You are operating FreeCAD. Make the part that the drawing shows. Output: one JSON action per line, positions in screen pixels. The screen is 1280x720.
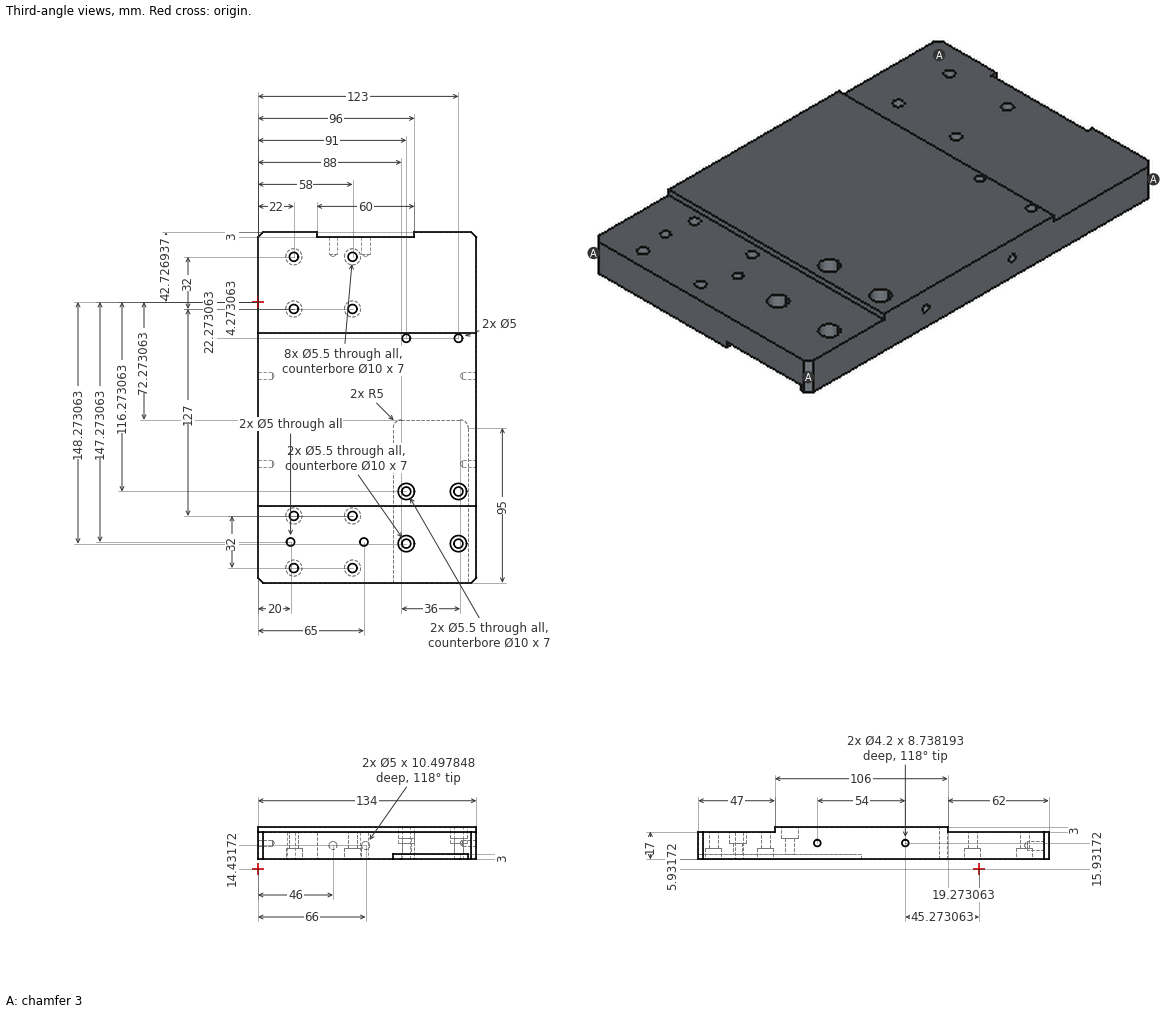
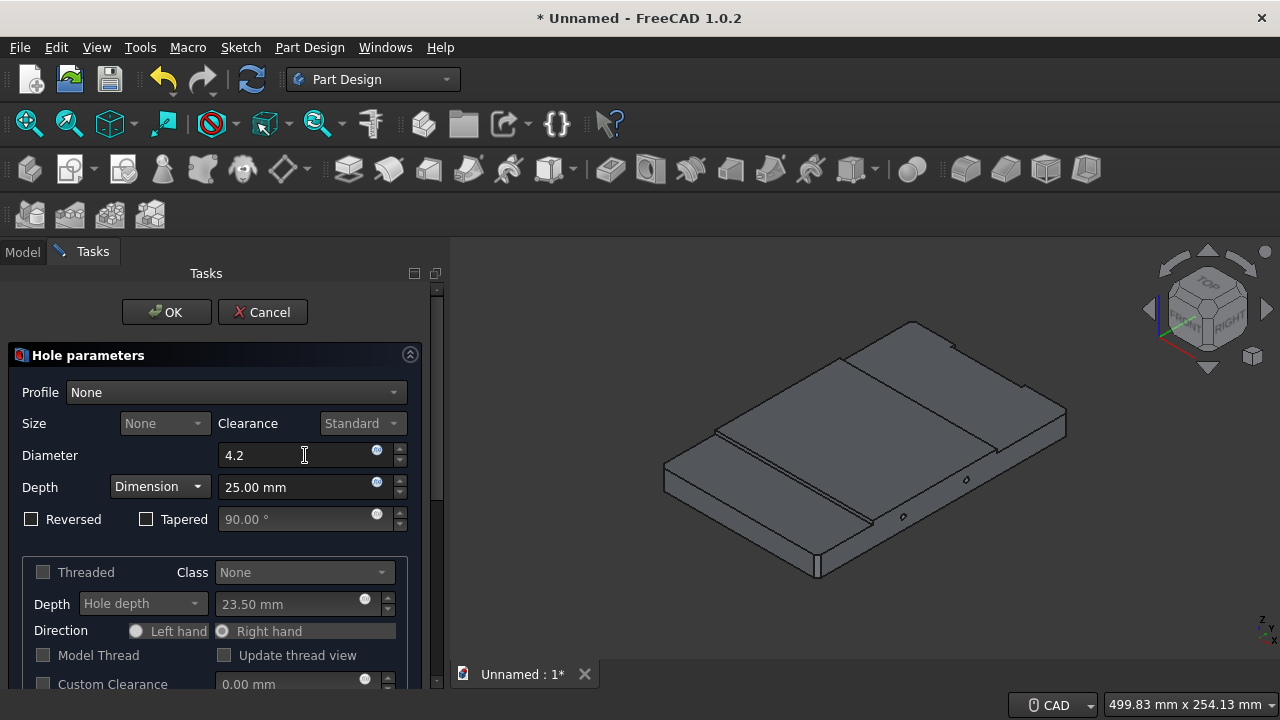
{"action": "triple_click", "coordinate": [305, 487]}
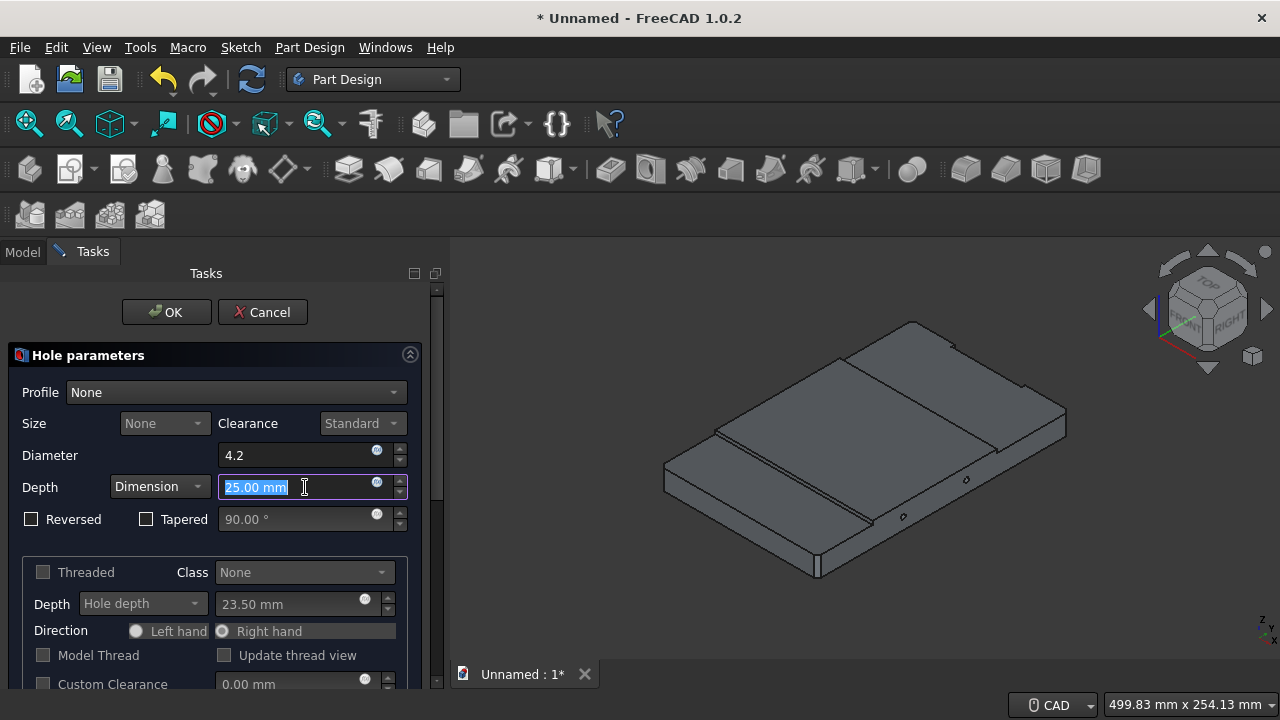
{"action": "type", "text": "8.738193"}
{"action": "key", "text": "Tab"}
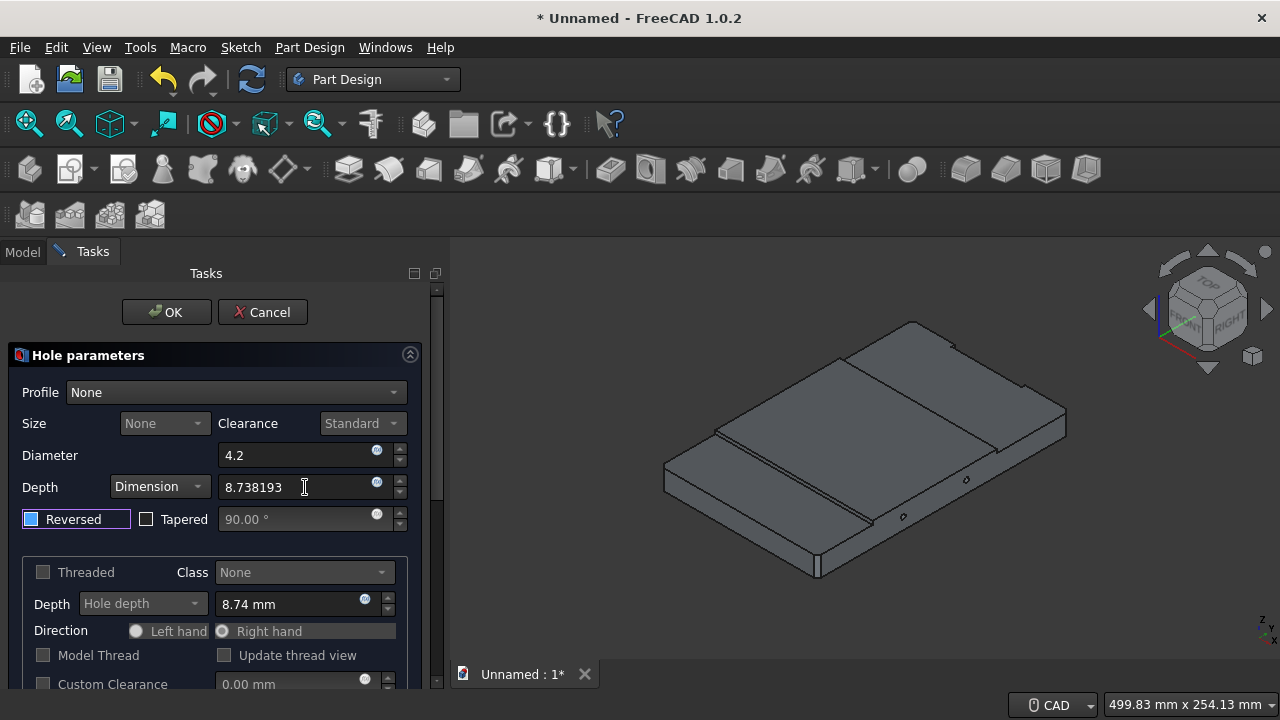
{"action": "left_click", "coordinate": [167, 312]}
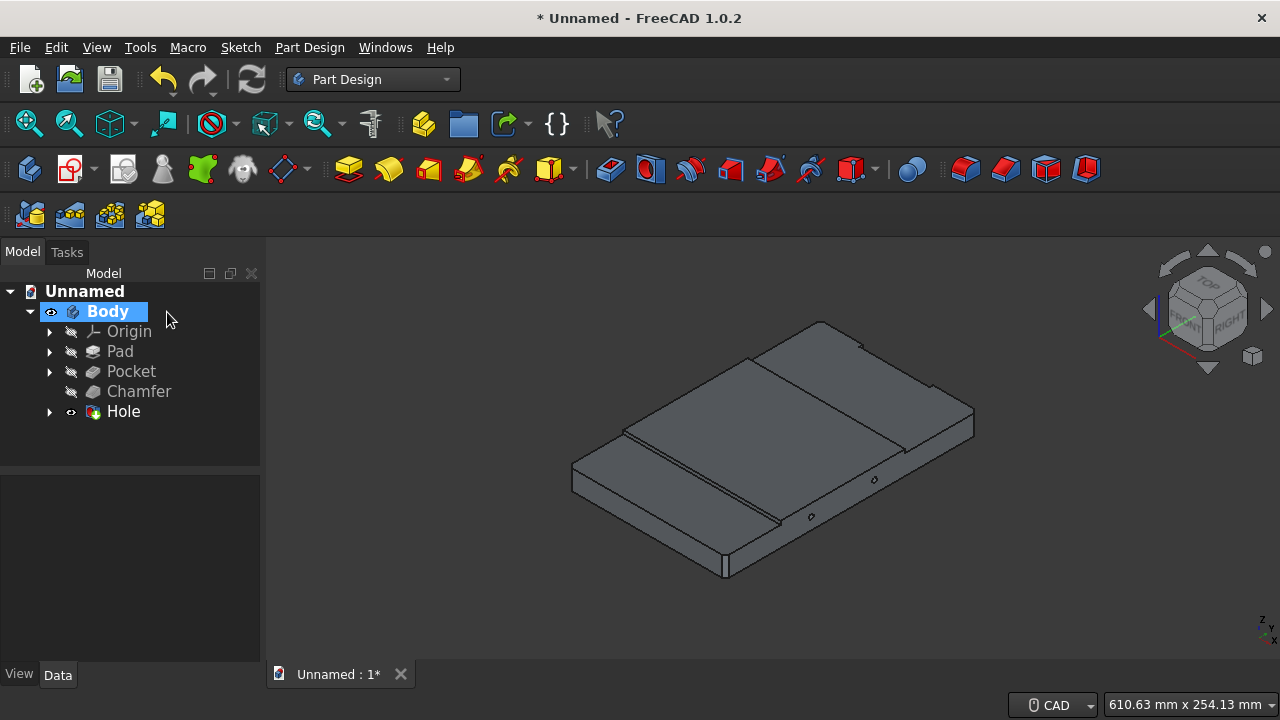
{"action": "key", "text": "6"}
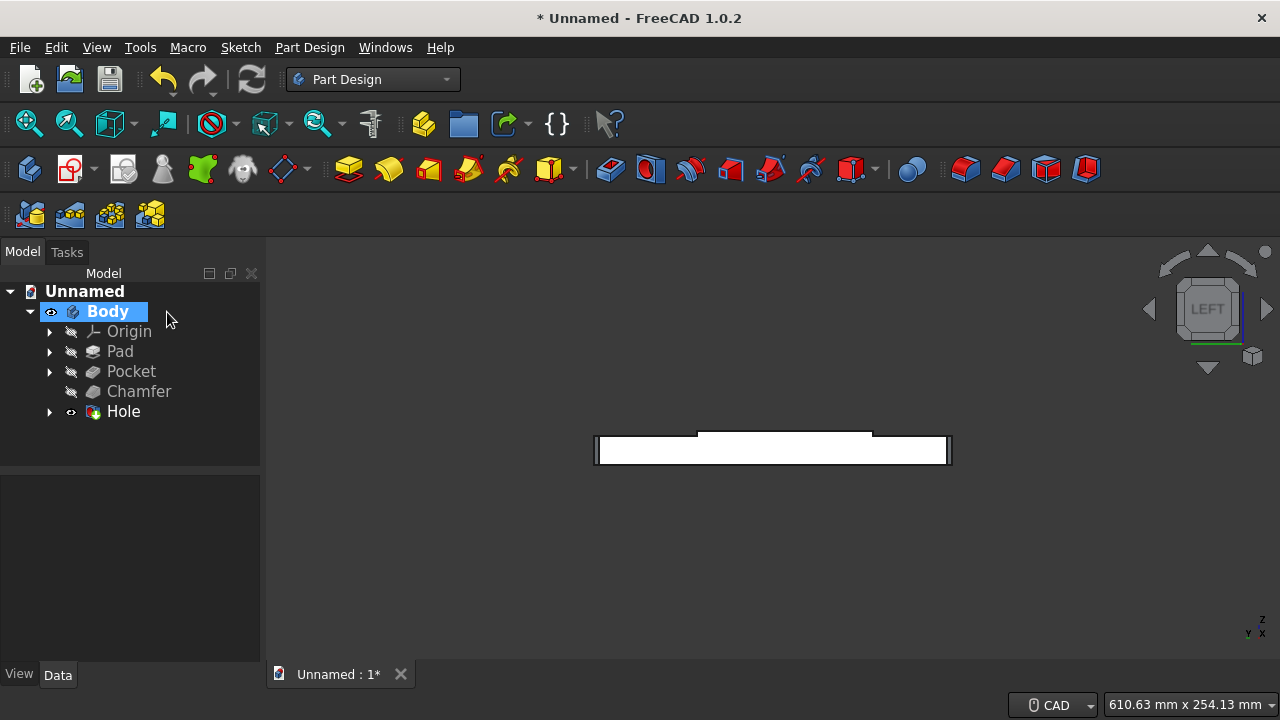
{"action": "left_click", "coordinate": [30, 124]}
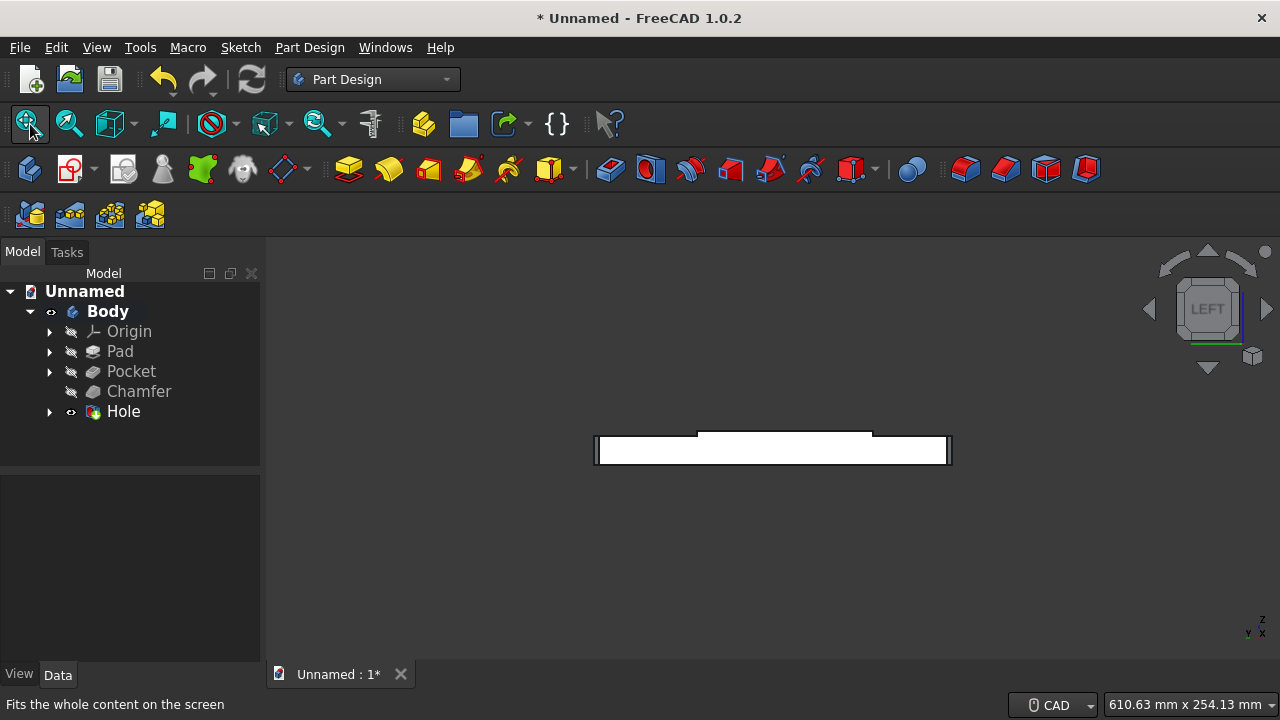
{"action": "left_click", "coordinate": [723, 447]}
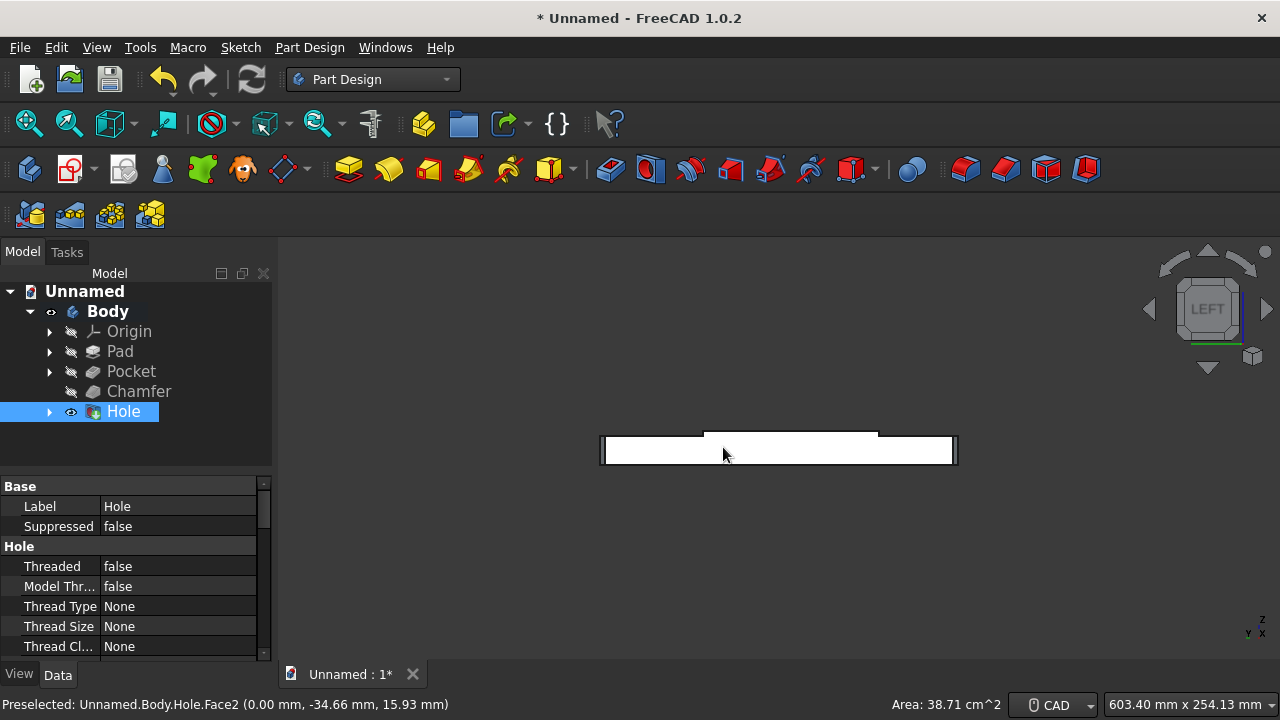
{"action": "left_click", "coordinate": [70, 170]}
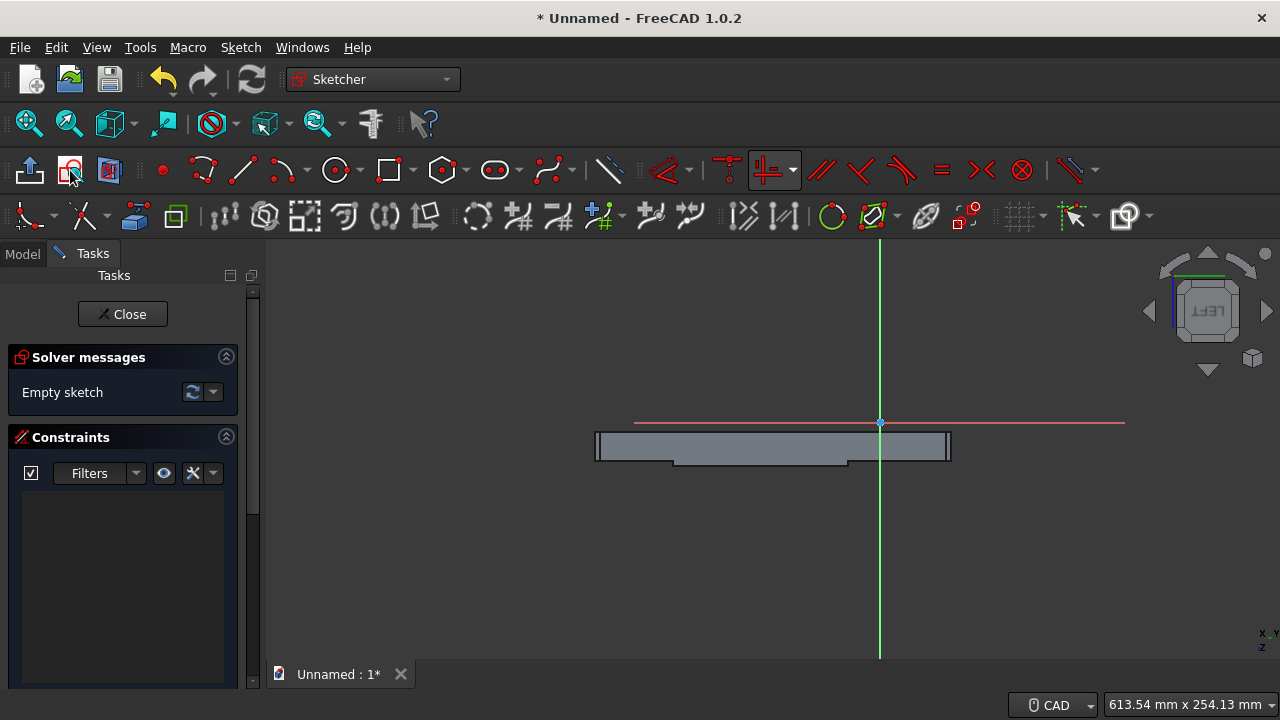
{"action": "scroll", "coordinate": [836, 433], "scroll_direction": "up", "scroll_amount": 6}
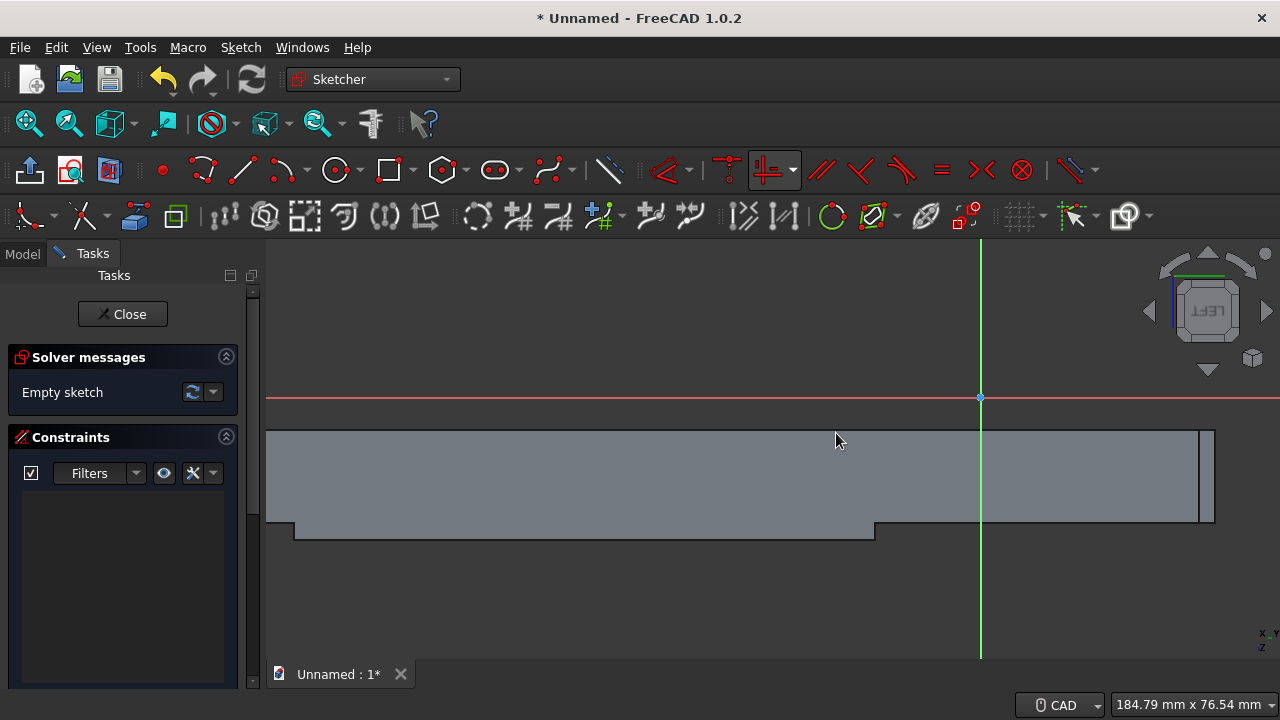
{"action": "left_click", "coordinate": [336, 170]}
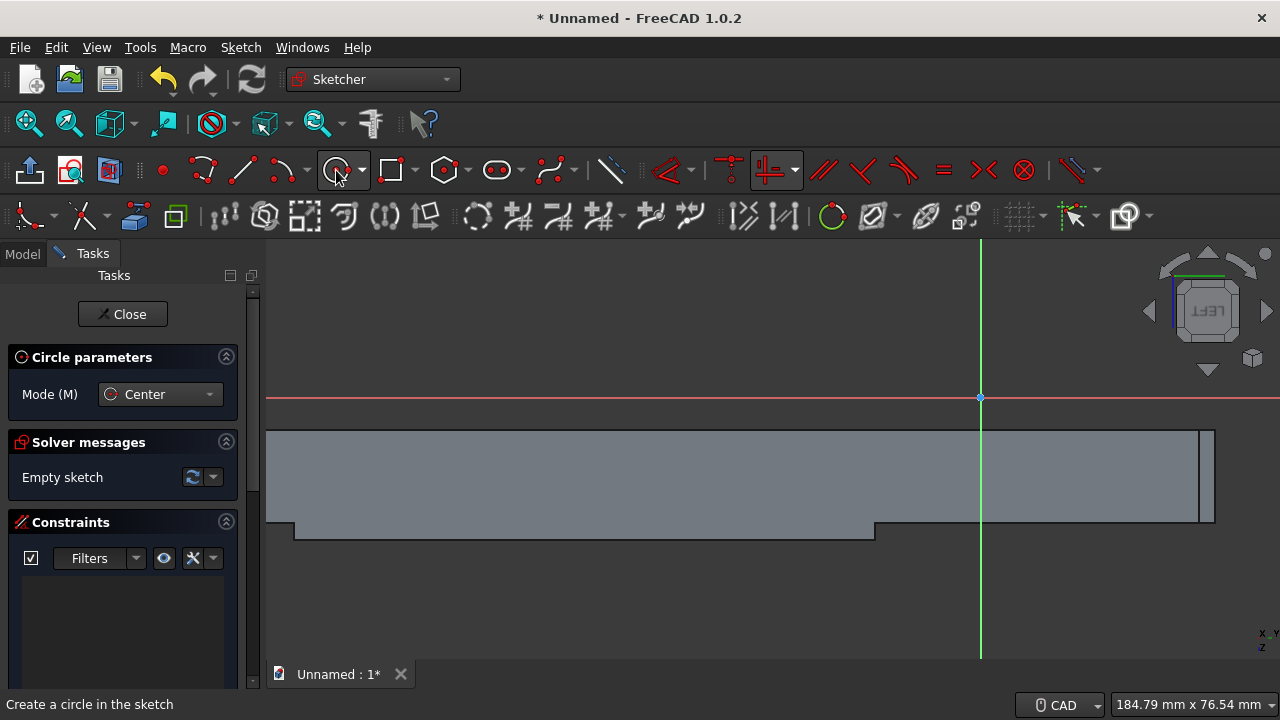
{"action": "scroll", "coordinate": [733, 485], "scroll_direction": "up", "scroll_amount": 4}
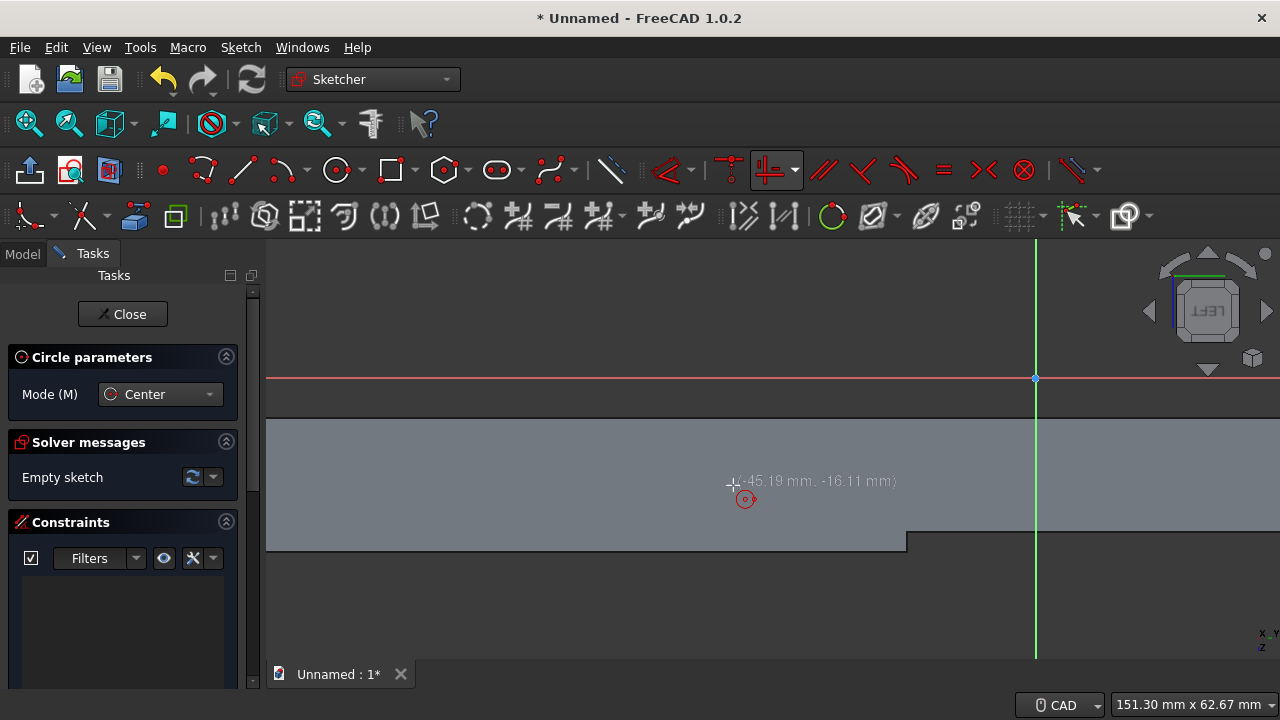
{"action": "left_click", "coordinate": [731, 484]}
{"action": "mouse_move", "coordinate": [750, 466]}